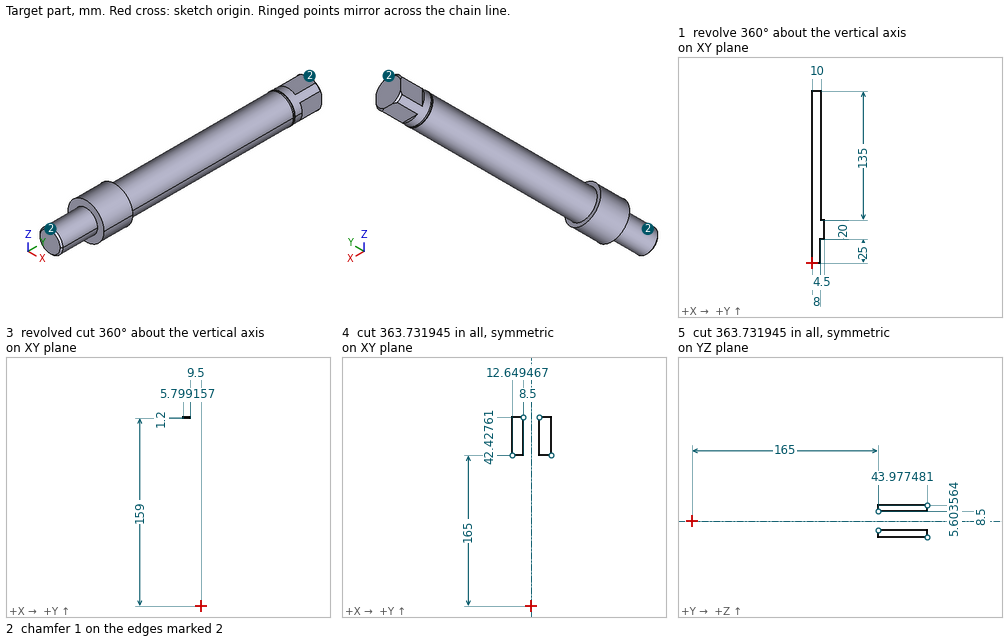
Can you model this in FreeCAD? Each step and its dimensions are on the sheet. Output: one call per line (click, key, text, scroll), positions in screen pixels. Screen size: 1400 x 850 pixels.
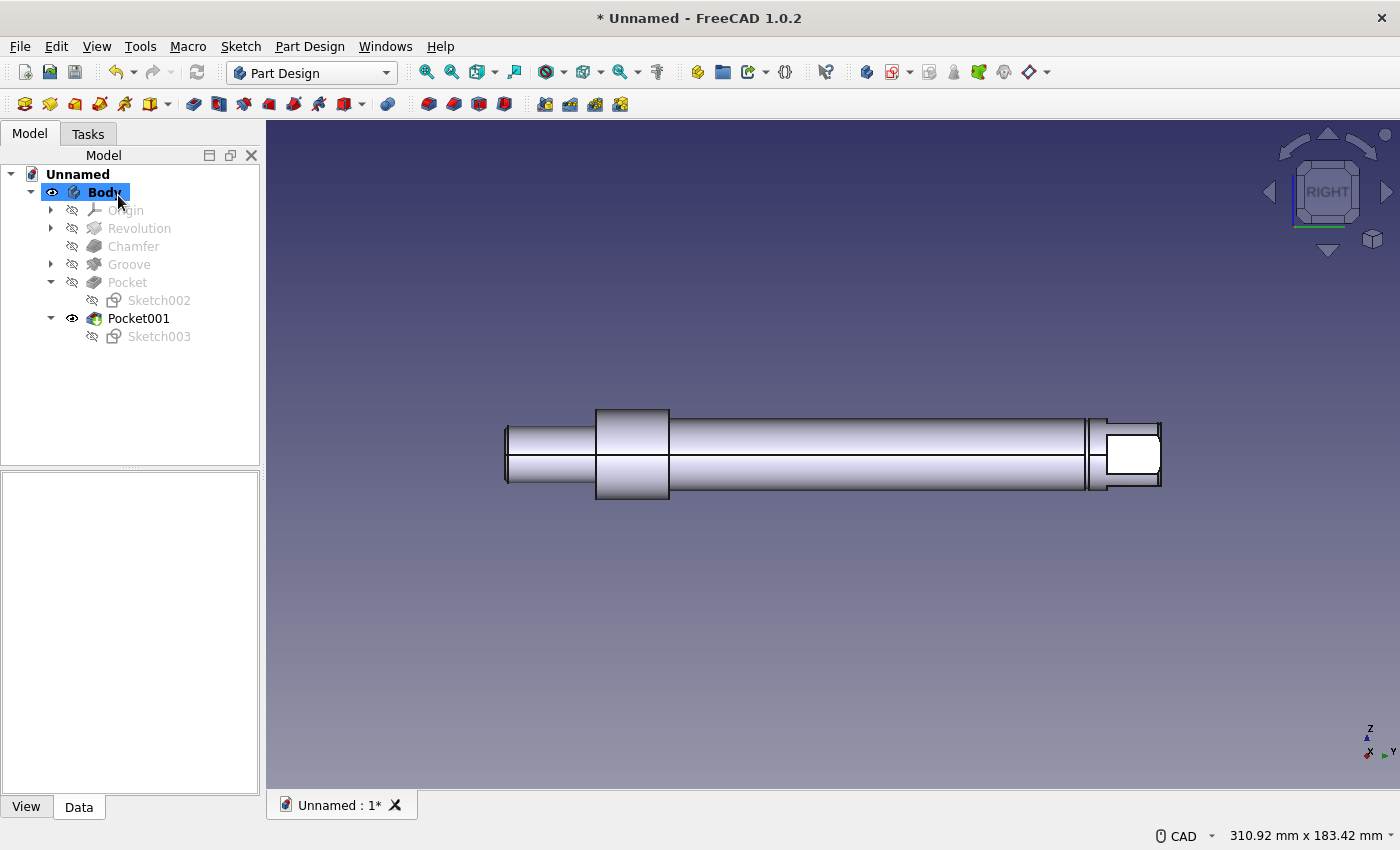
key(0)